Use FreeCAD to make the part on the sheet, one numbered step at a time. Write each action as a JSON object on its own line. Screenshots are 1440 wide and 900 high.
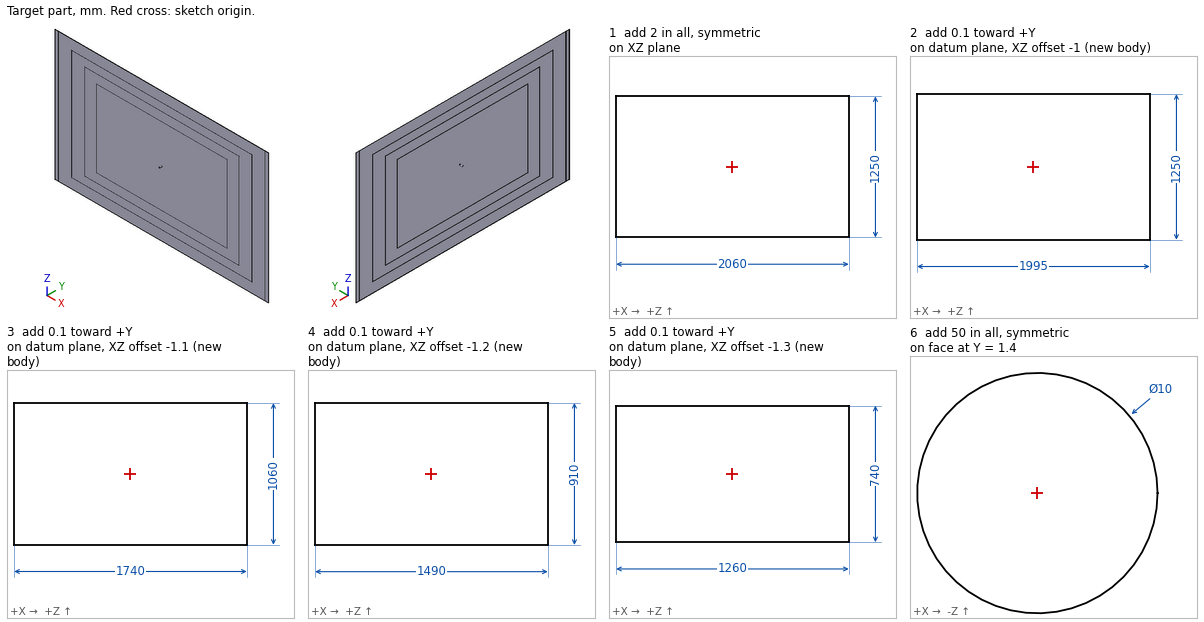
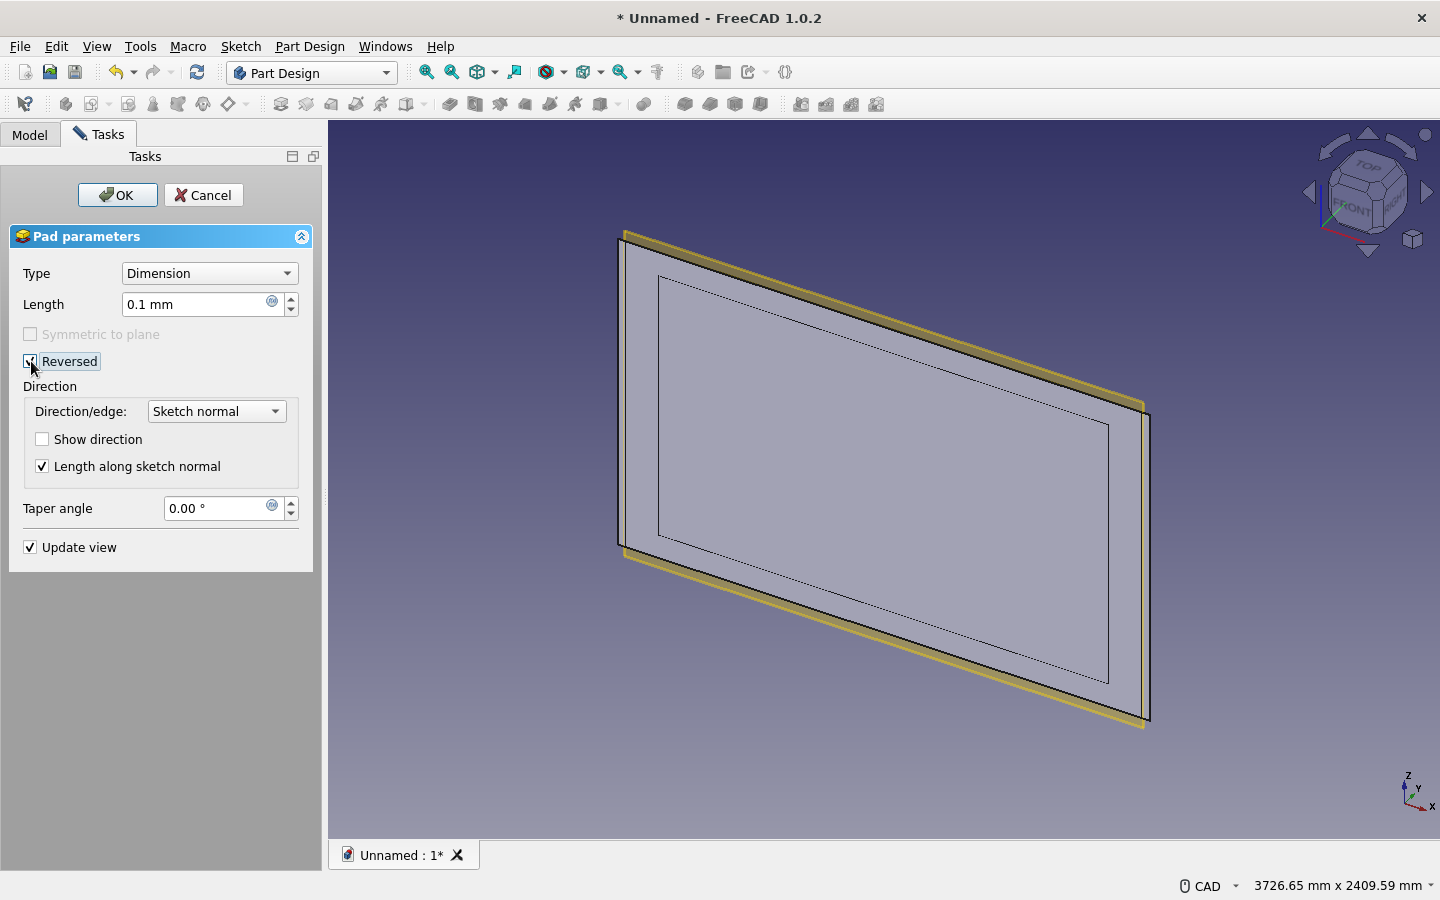
{"action": "left_click", "coordinate": [118, 195]}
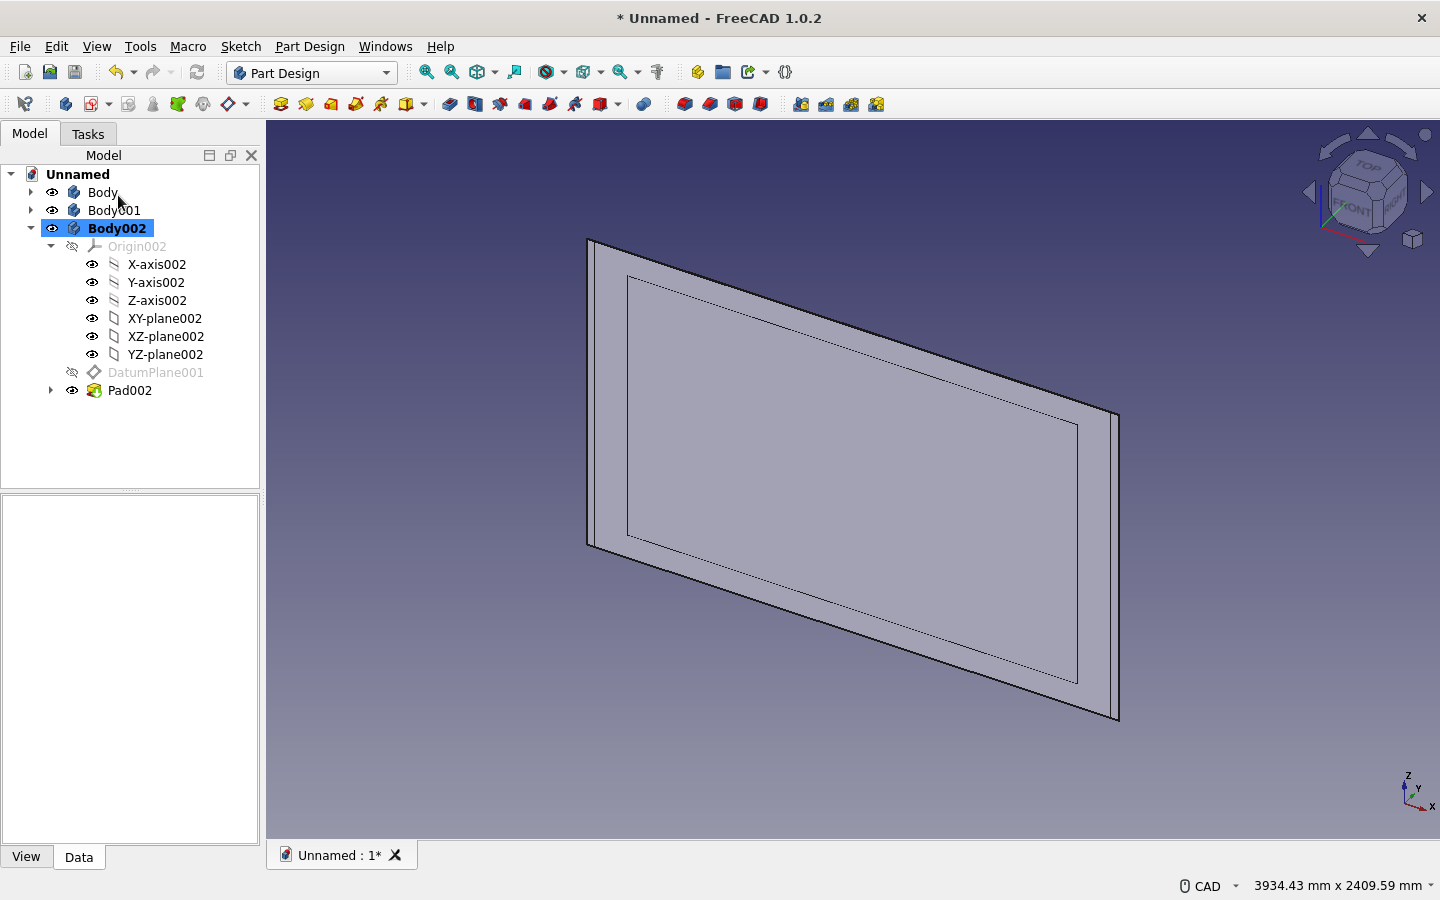
{"action": "left_click", "coordinate": [66, 104]}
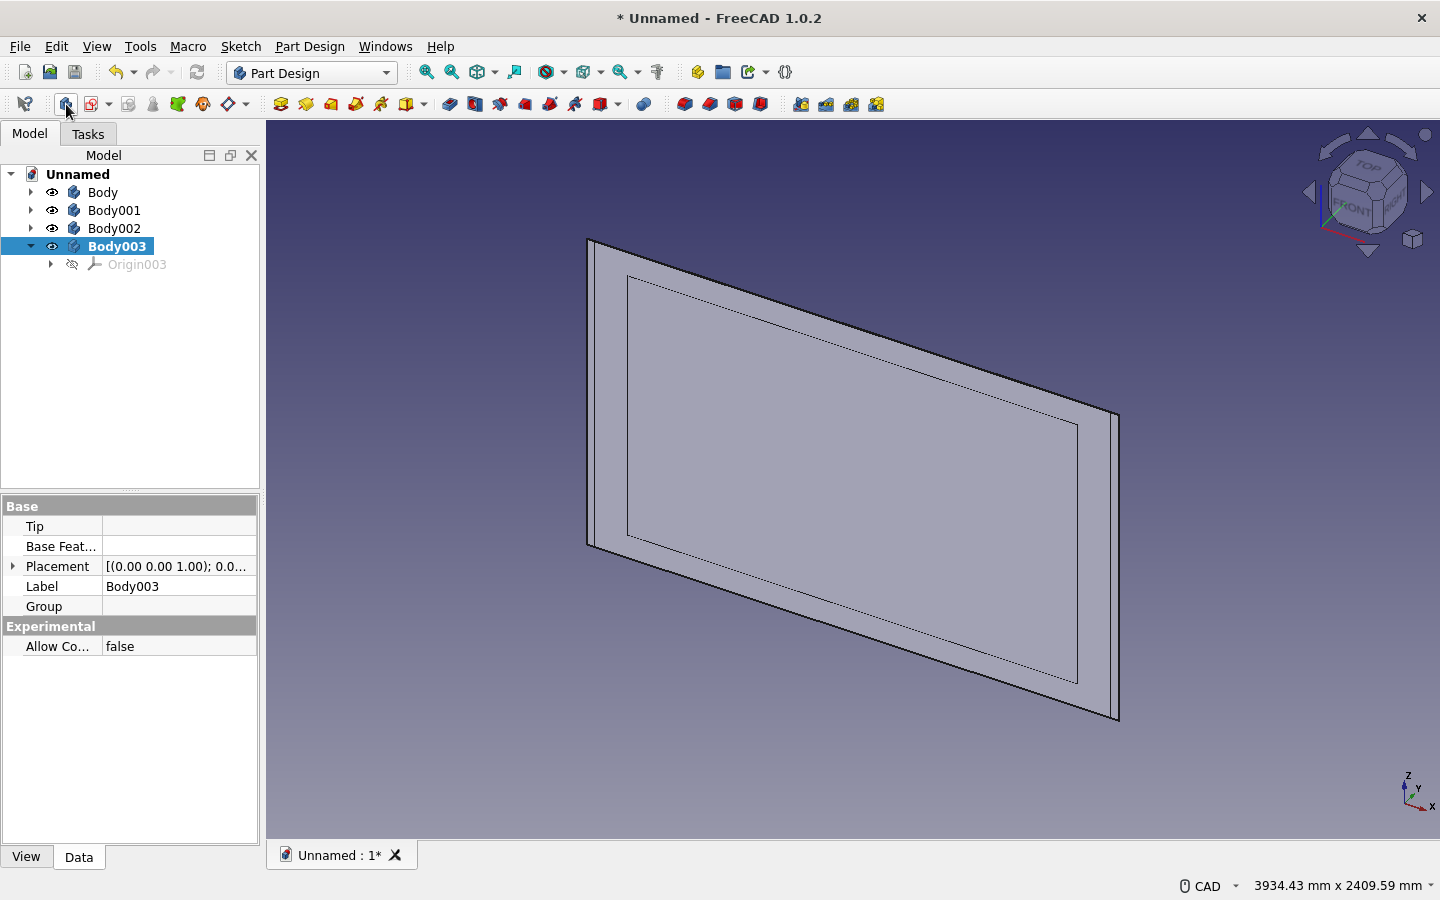
{"action": "left_click", "coordinate": [51, 264]}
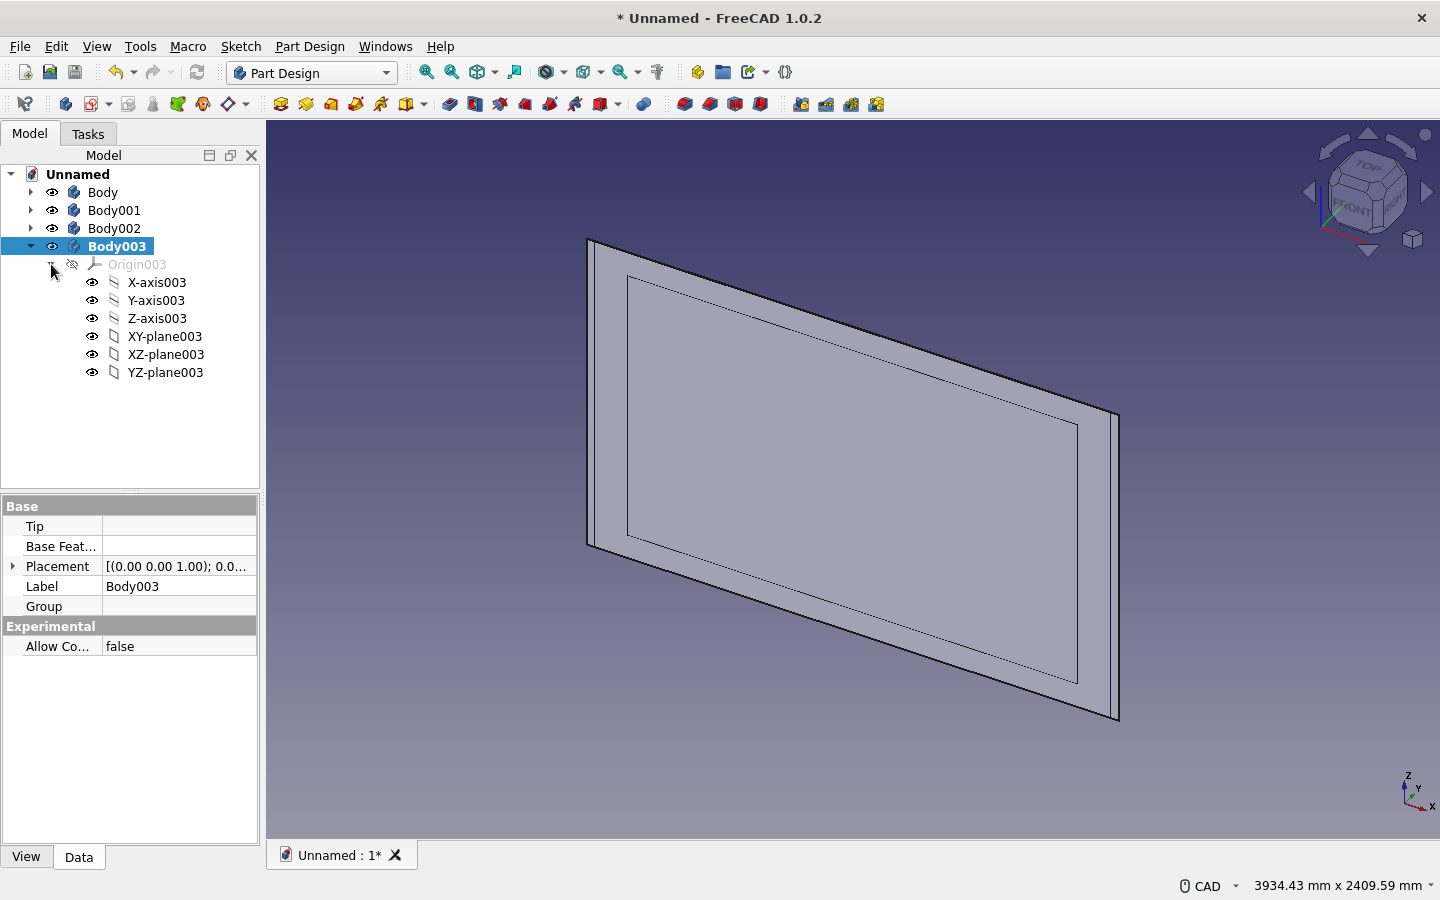
{"action": "left_click", "coordinate": [137, 354]}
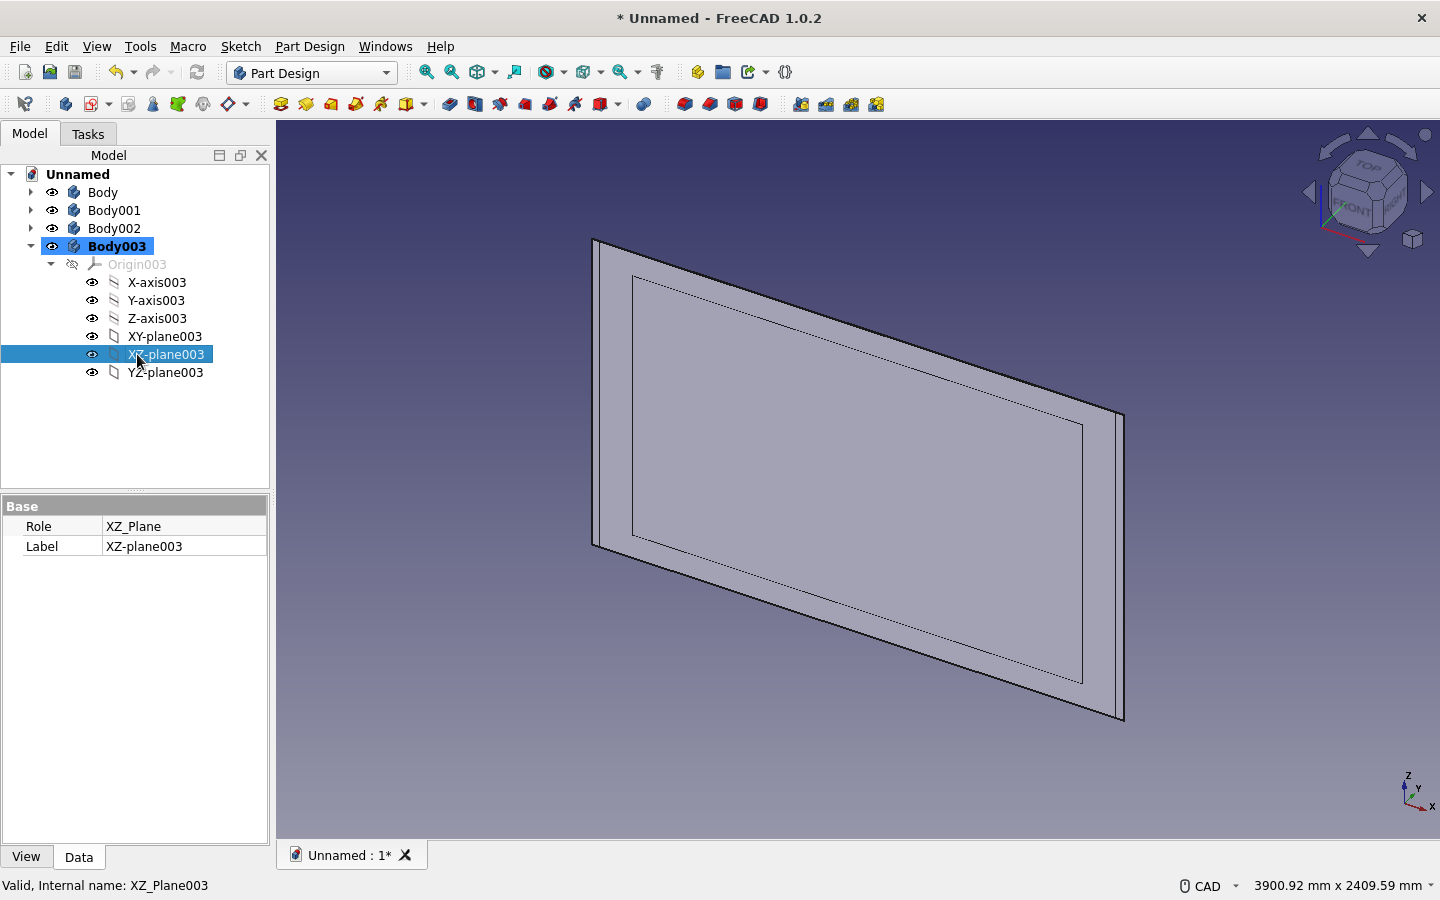
{"action": "left_click", "coordinate": [228, 104]}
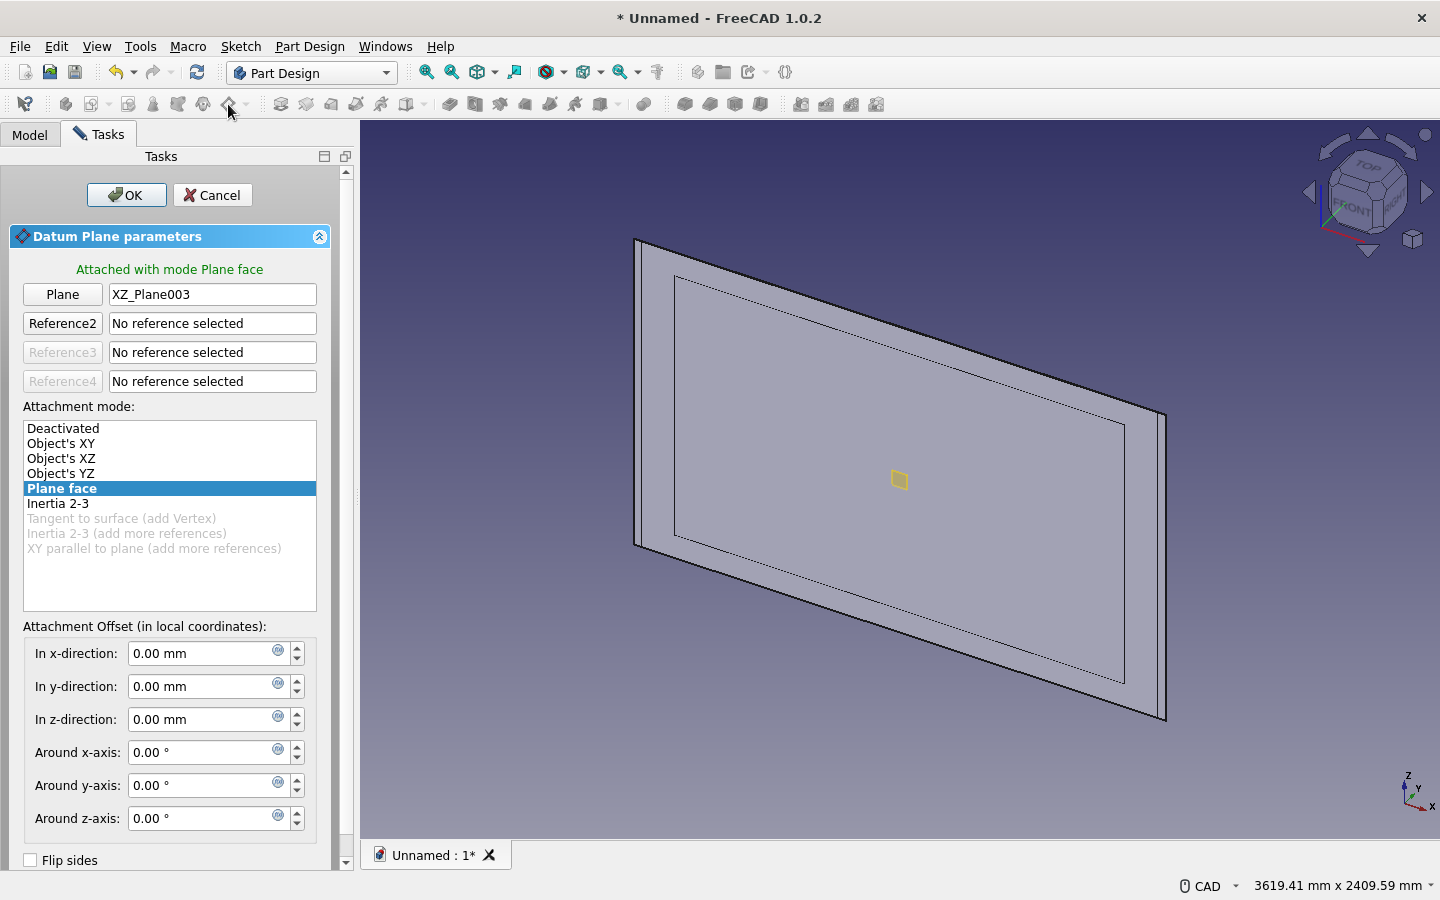
{"action": "triple_click", "coordinate": [210, 720]}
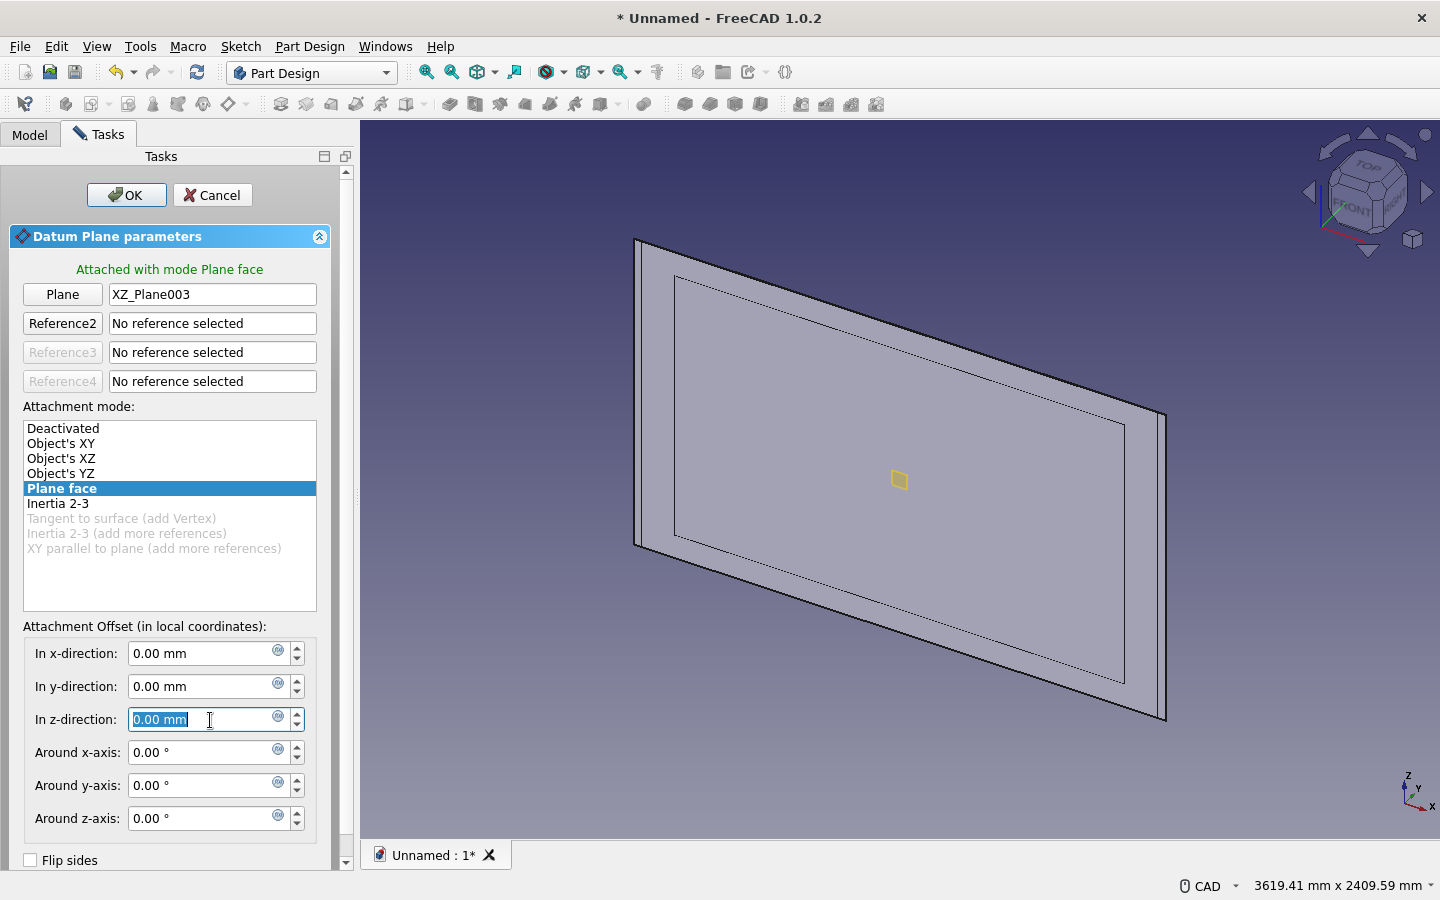
{"action": "type", "text": "-1.2"}
{"action": "key", "text": "Tab"}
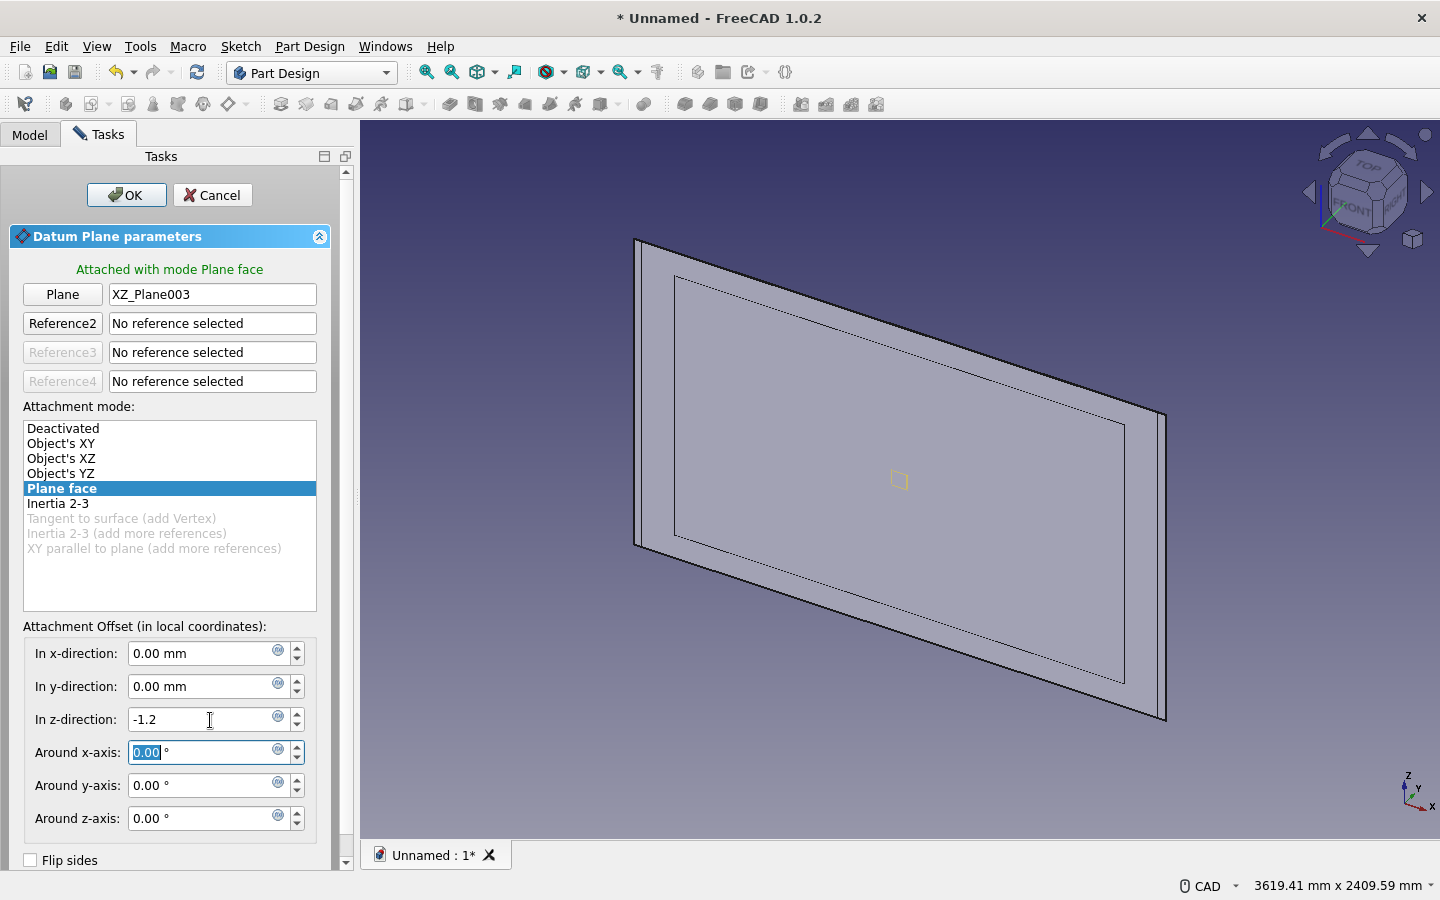
{"action": "left_click", "coordinate": [127, 195]}